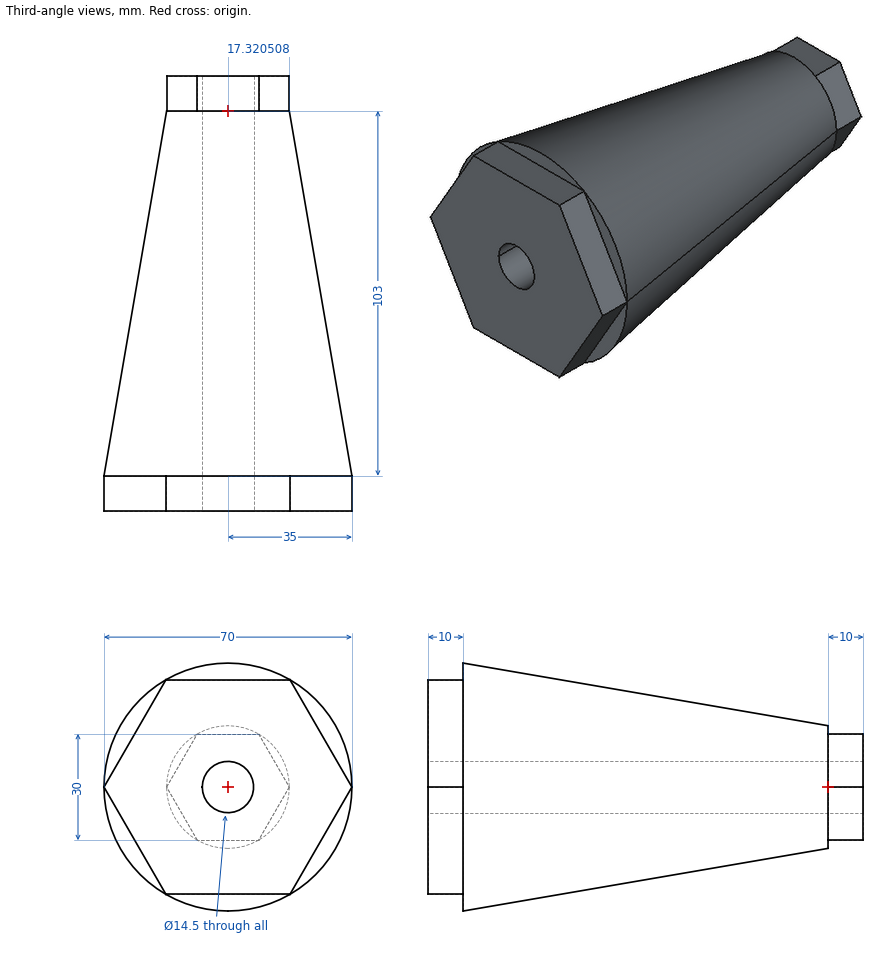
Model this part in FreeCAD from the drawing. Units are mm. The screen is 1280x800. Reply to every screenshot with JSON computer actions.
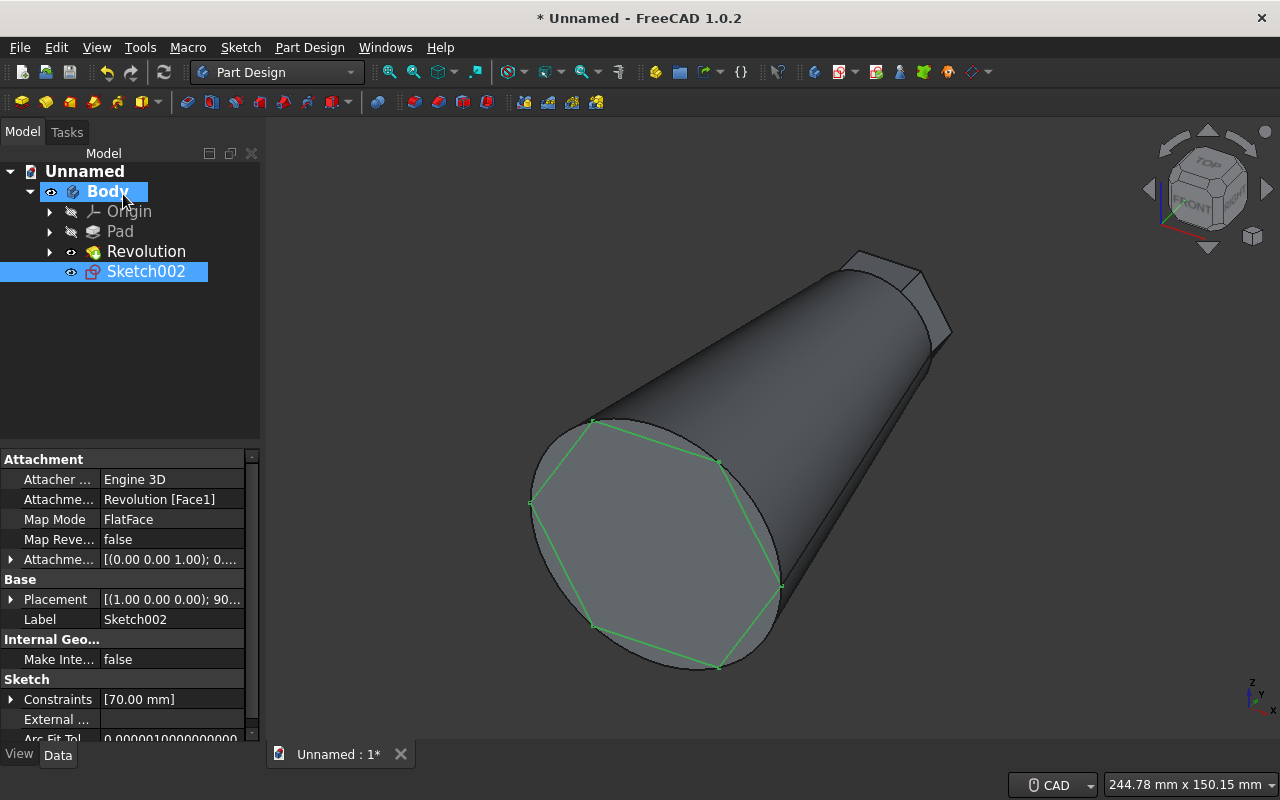
{"action": "left_click", "coordinate": [22, 102]}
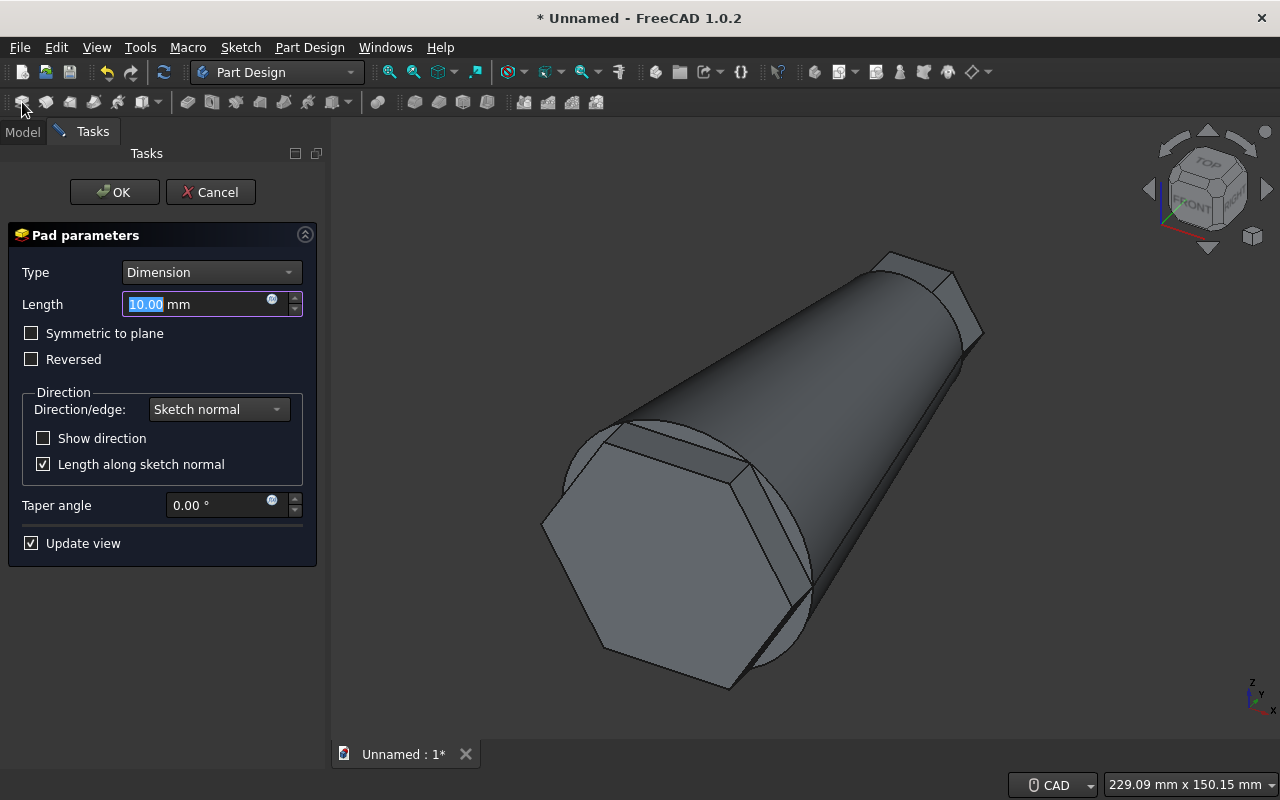
{"action": "type", "text": "10"}
{"action": "key", "text": "Tab"}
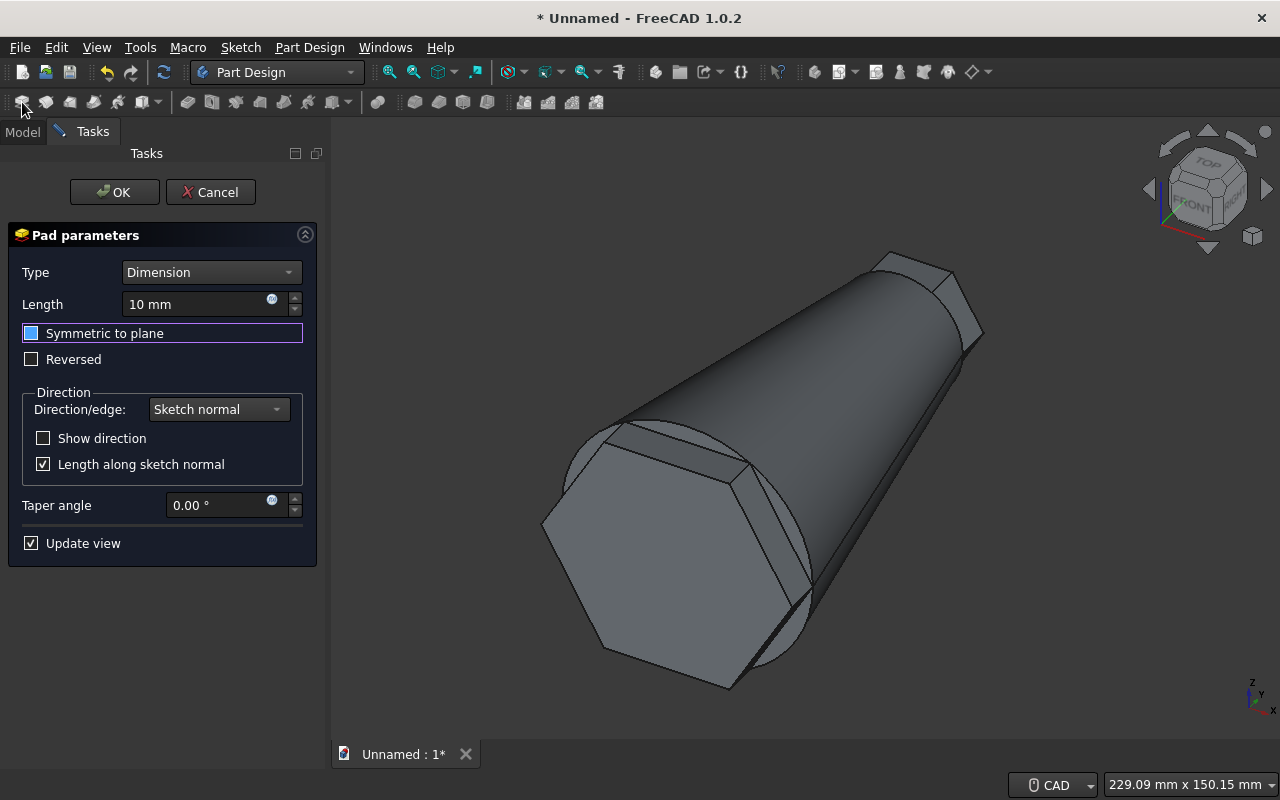
{"action": "left_click", "coordinate": [115, 192]}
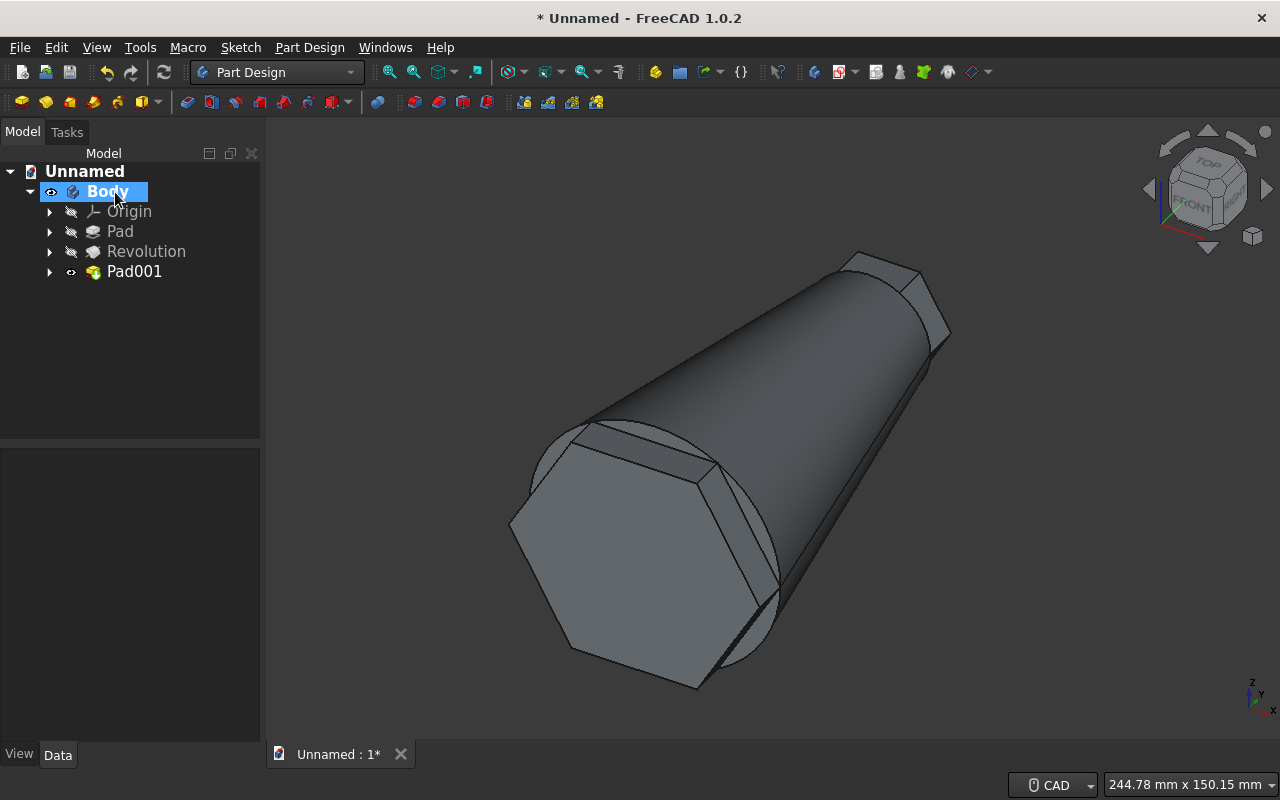
{"action": "key", "text": "4"}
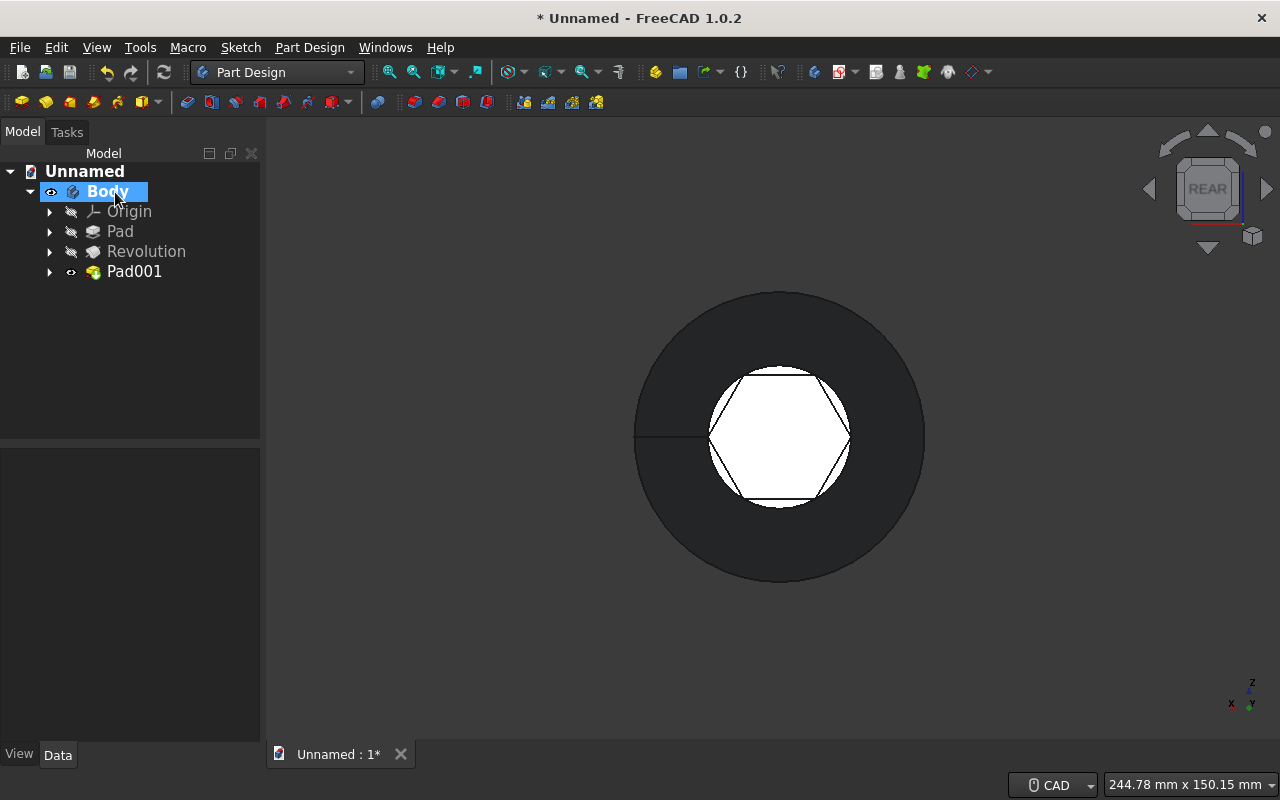
{"action": "left_click", "coordinate": [779, 436]}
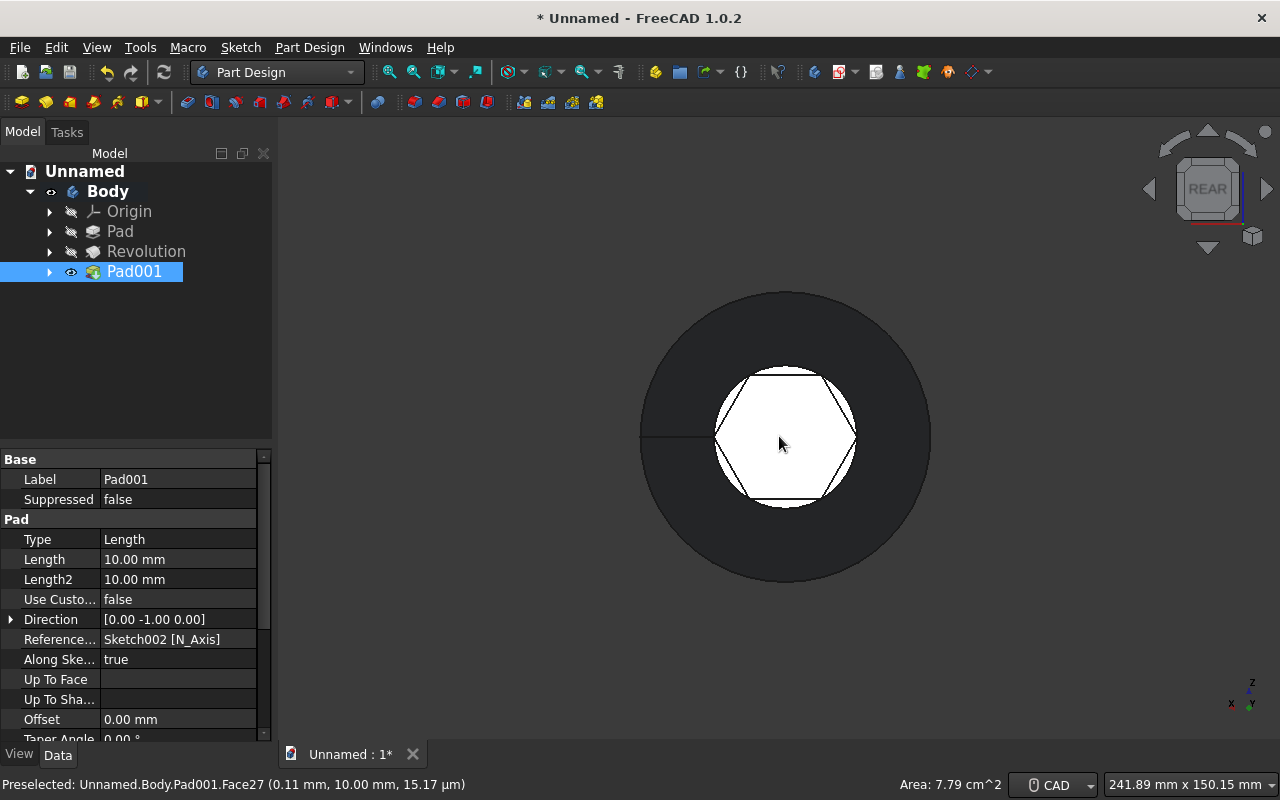
{"action": "left_click", "coordinate": [840, 72]}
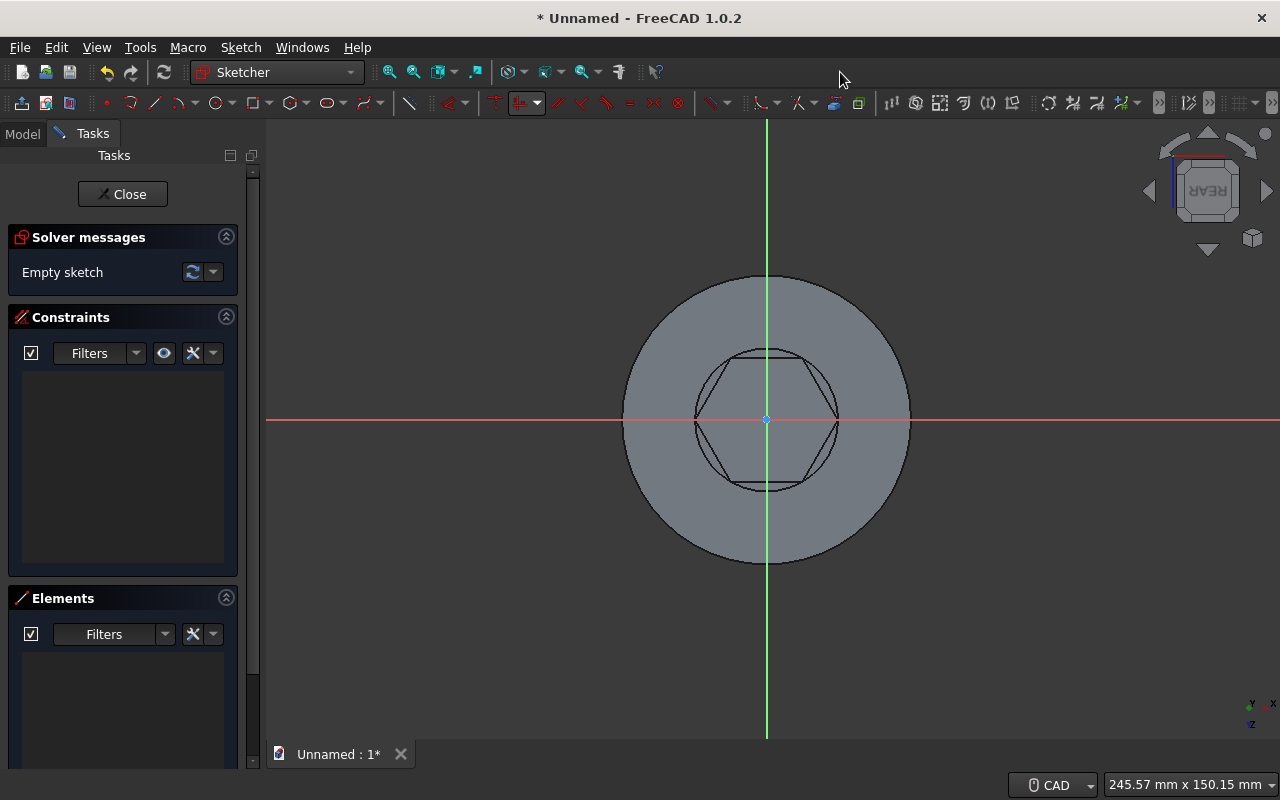
{"action": "scroll", "coordinate": [779, 418], "scroll_direction": "up", "scroll_amount": 9}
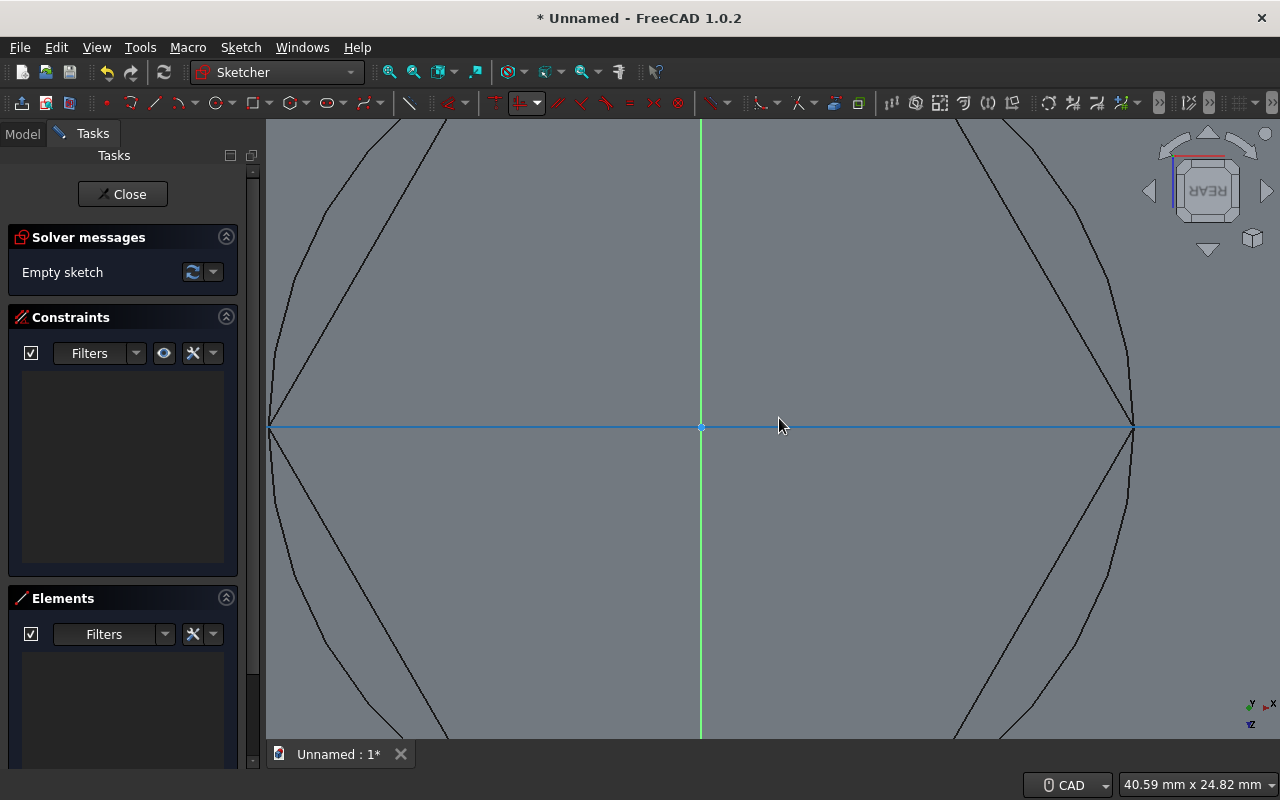
{"action": "left_click", "coordinate": [216, 104]}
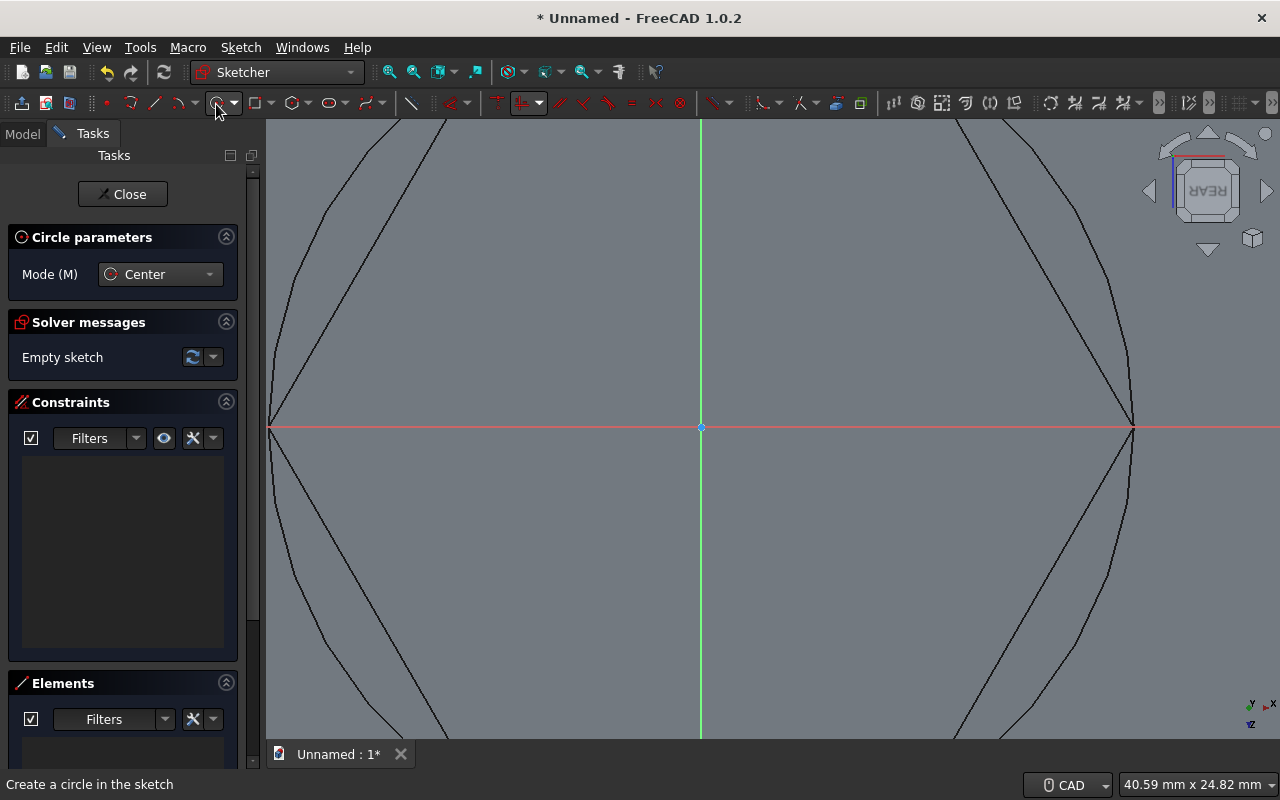
{"action": "left_click", "coordinate": [701, 427]}
{"action": "left_click", "coordinate": [829, 299]}
{"action": "key", "text": "Escape"}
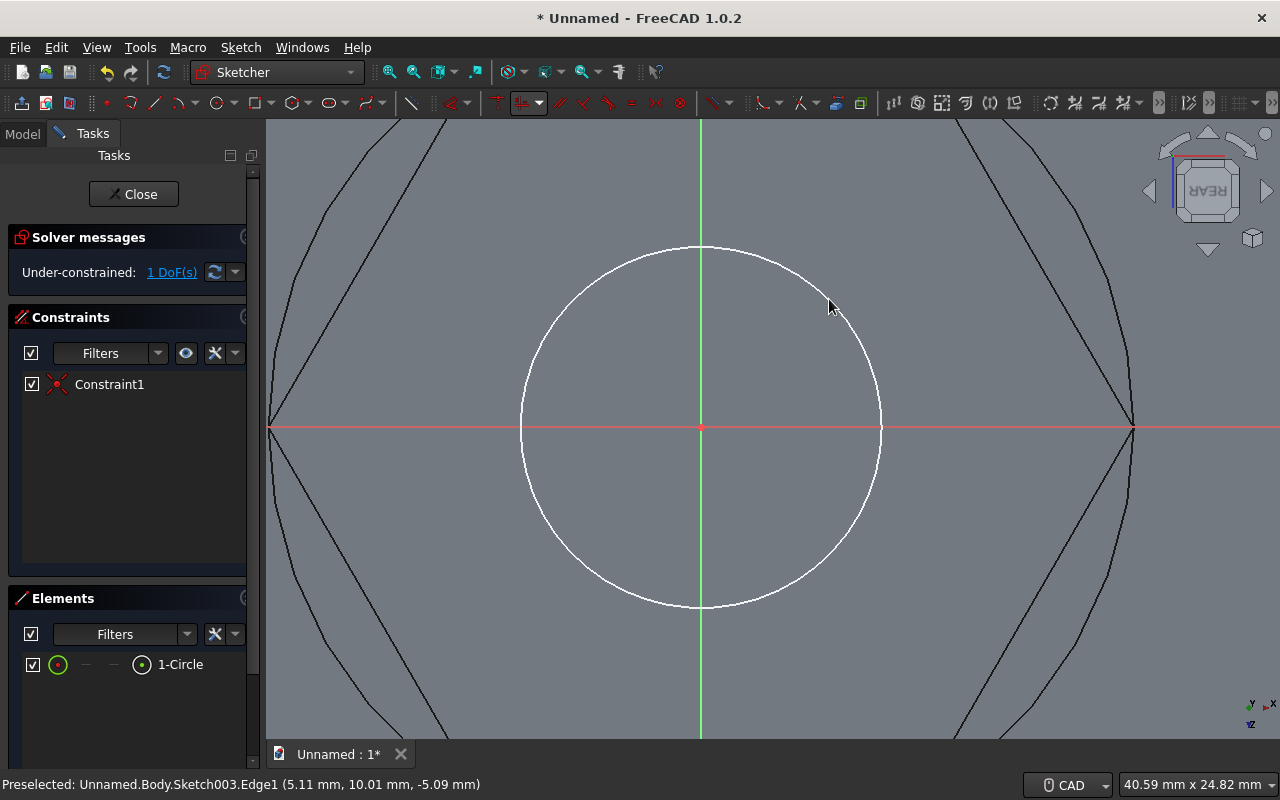
{"action": "left_click", "coordinate": [450, 104]}